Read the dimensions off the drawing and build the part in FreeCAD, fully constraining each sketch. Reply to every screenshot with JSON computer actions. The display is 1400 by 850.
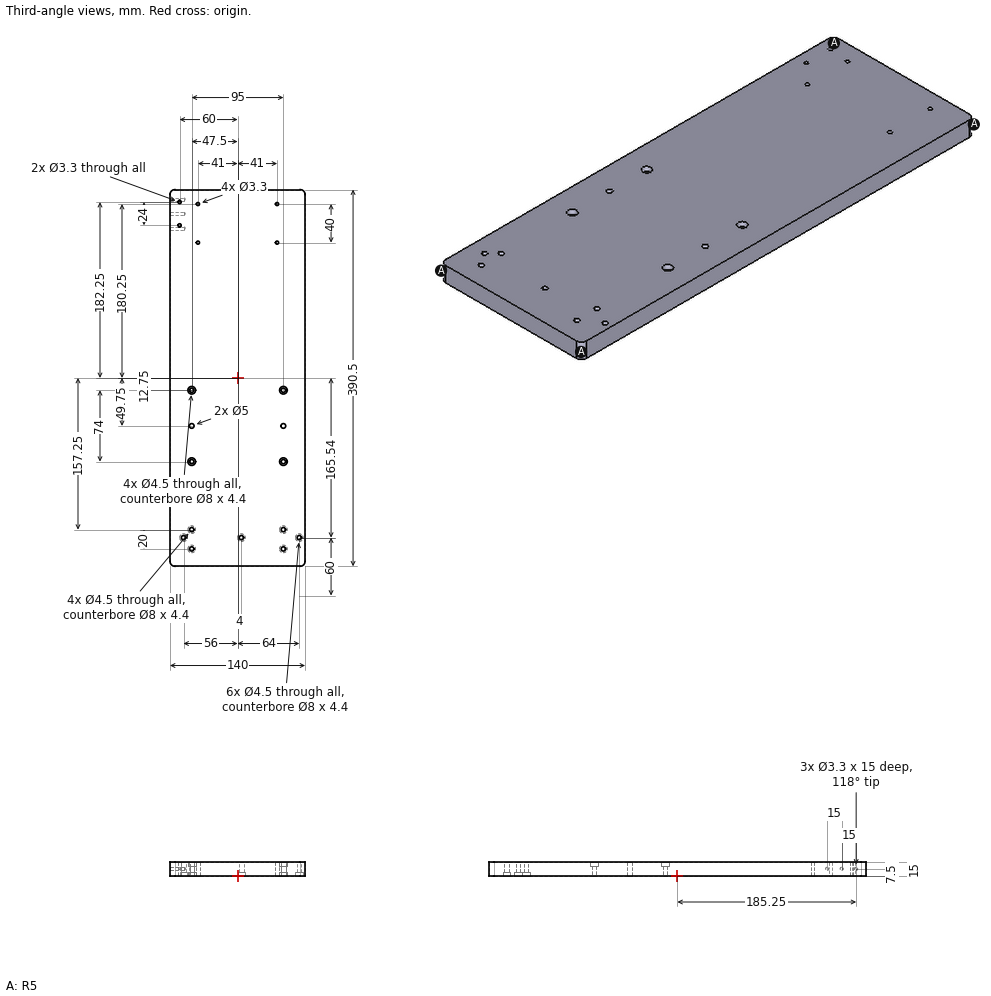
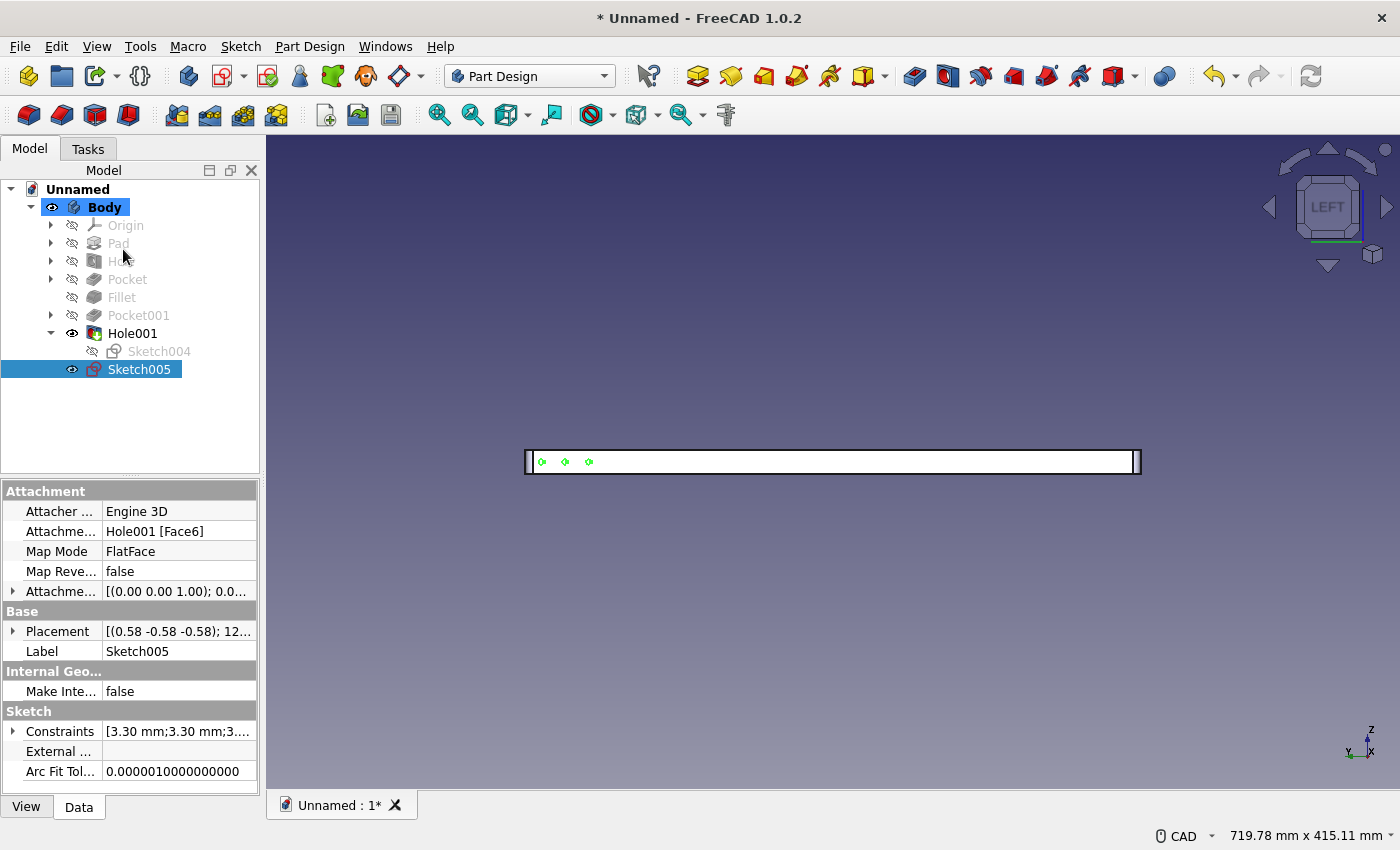
{"action": "left_click", "coordinate": [948, 76]}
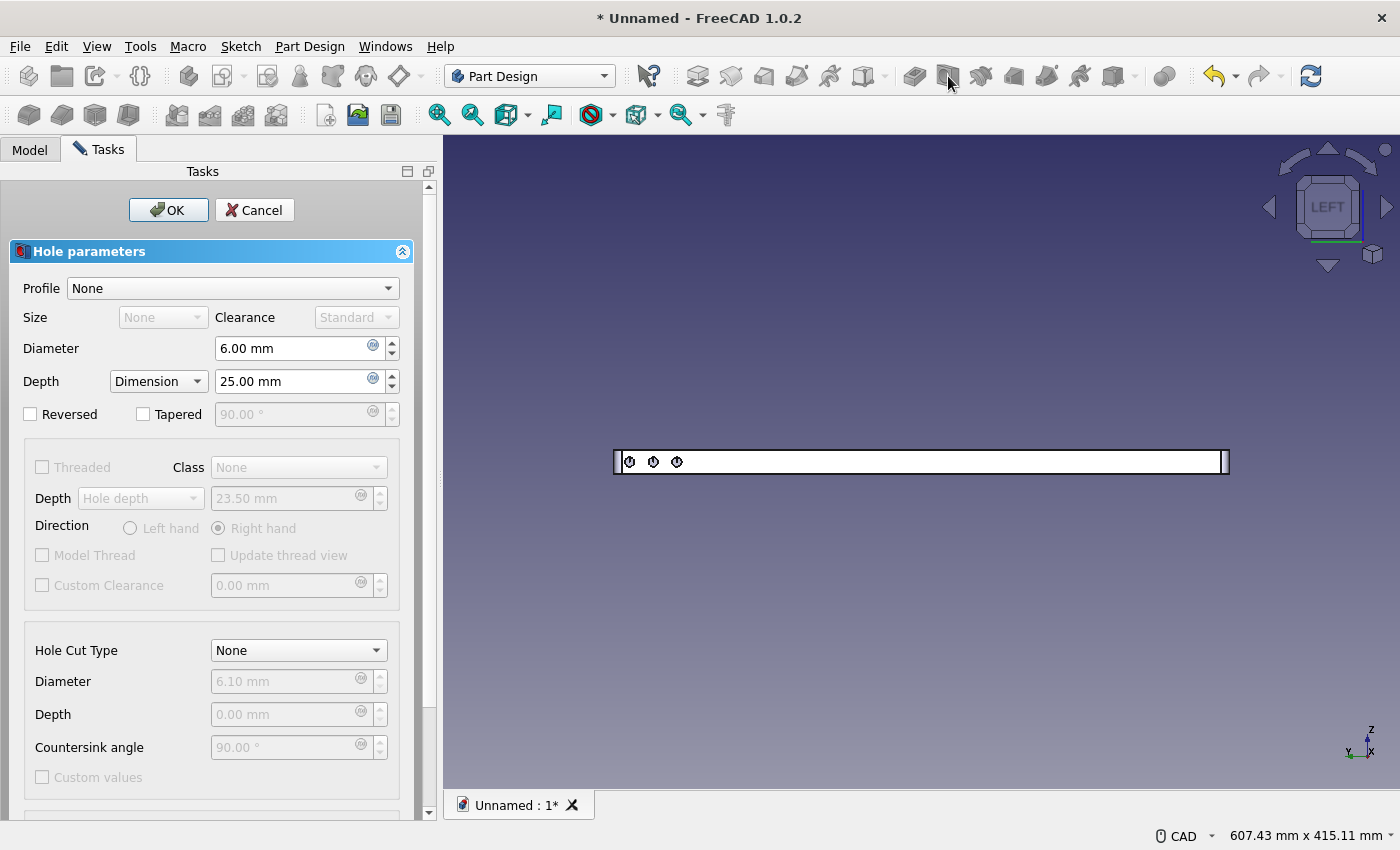
{"action": "triple_click", "coordinate": [300, 348]}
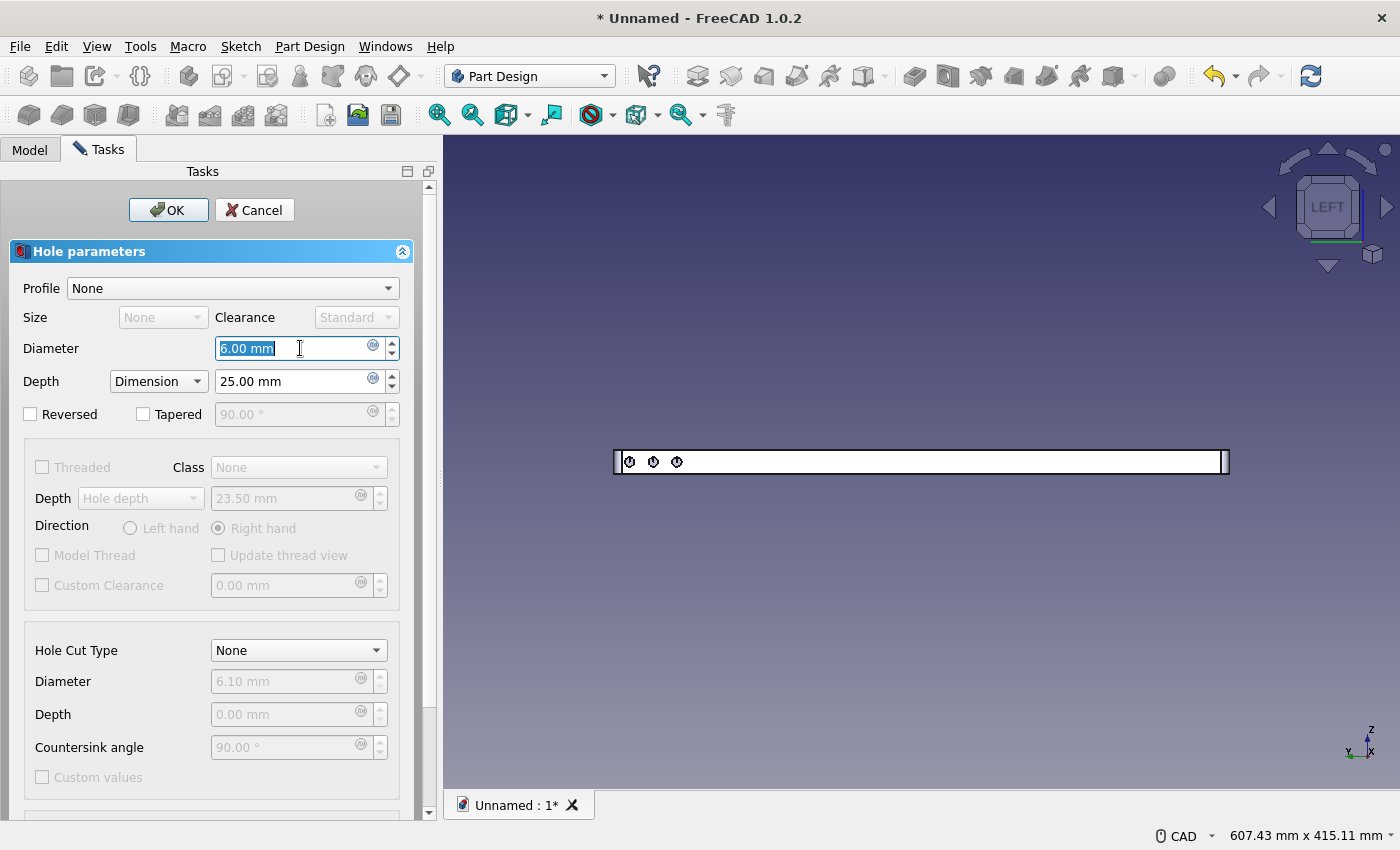
{"action": "type", "text": "3.3"}
{"action": "key", "text": "Tab"}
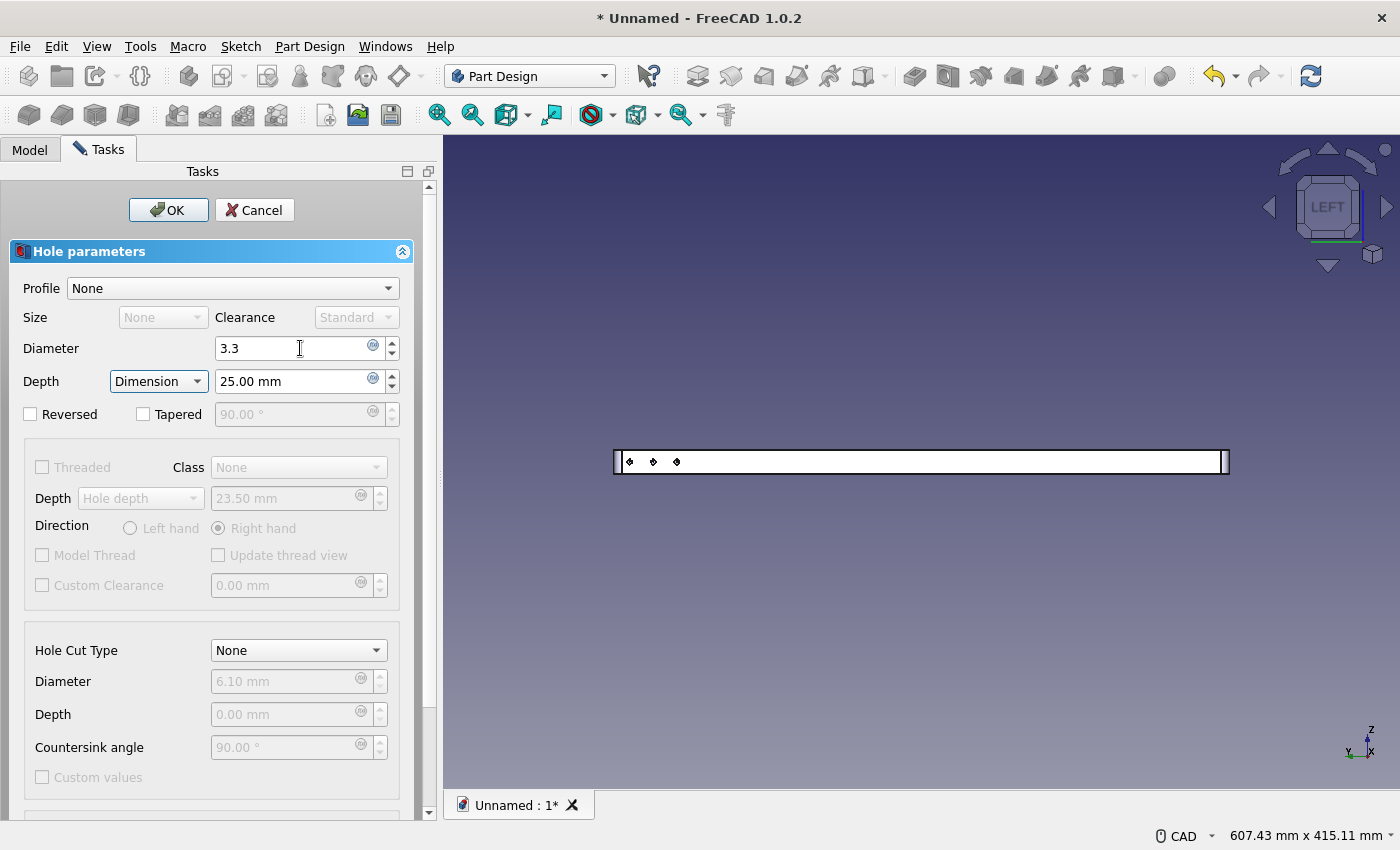
{"action": "triple_click", "coordinate": [300, 382]}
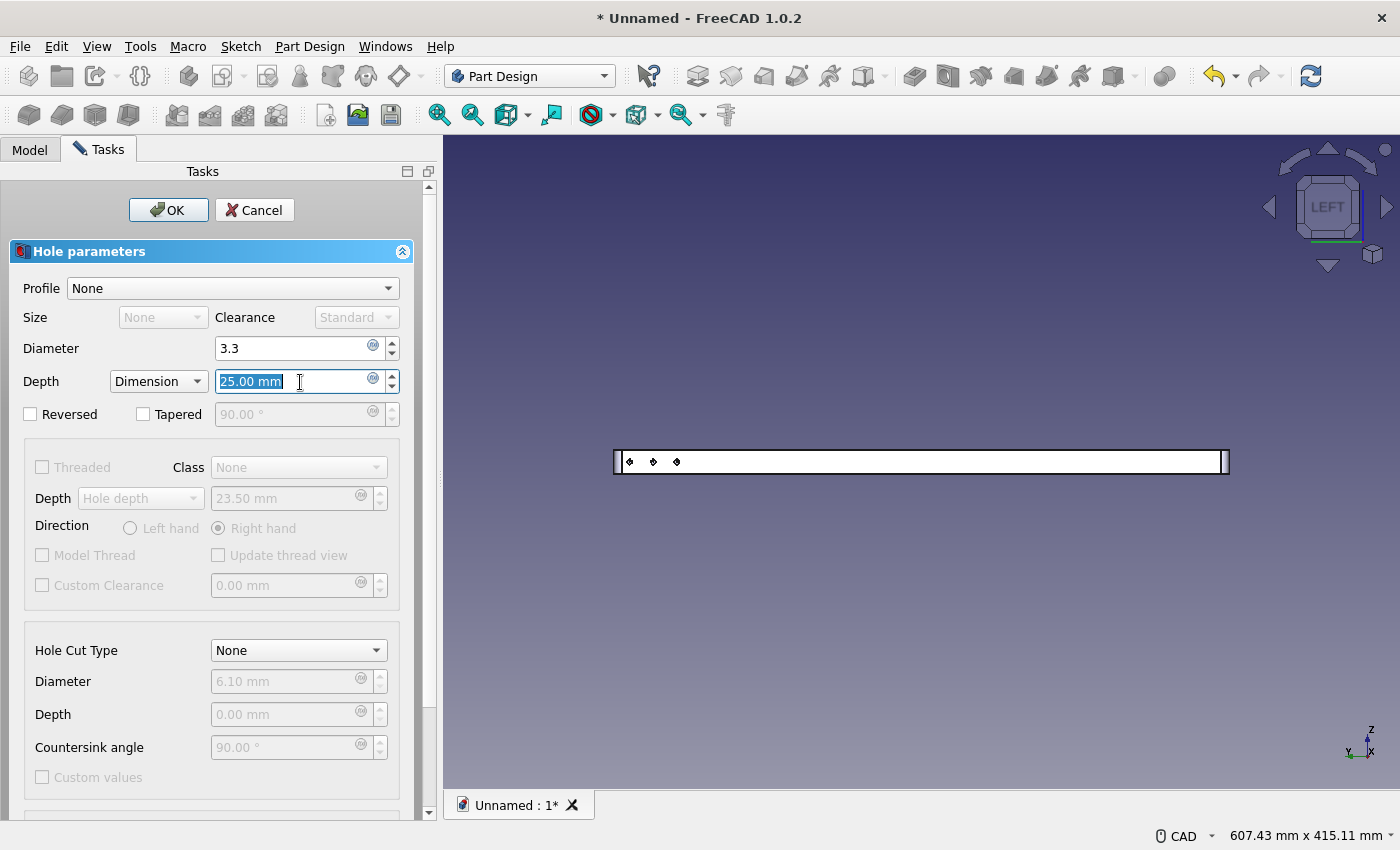
{"action": "type", "text": "15"}
{"action": "key", "text": "Tab"}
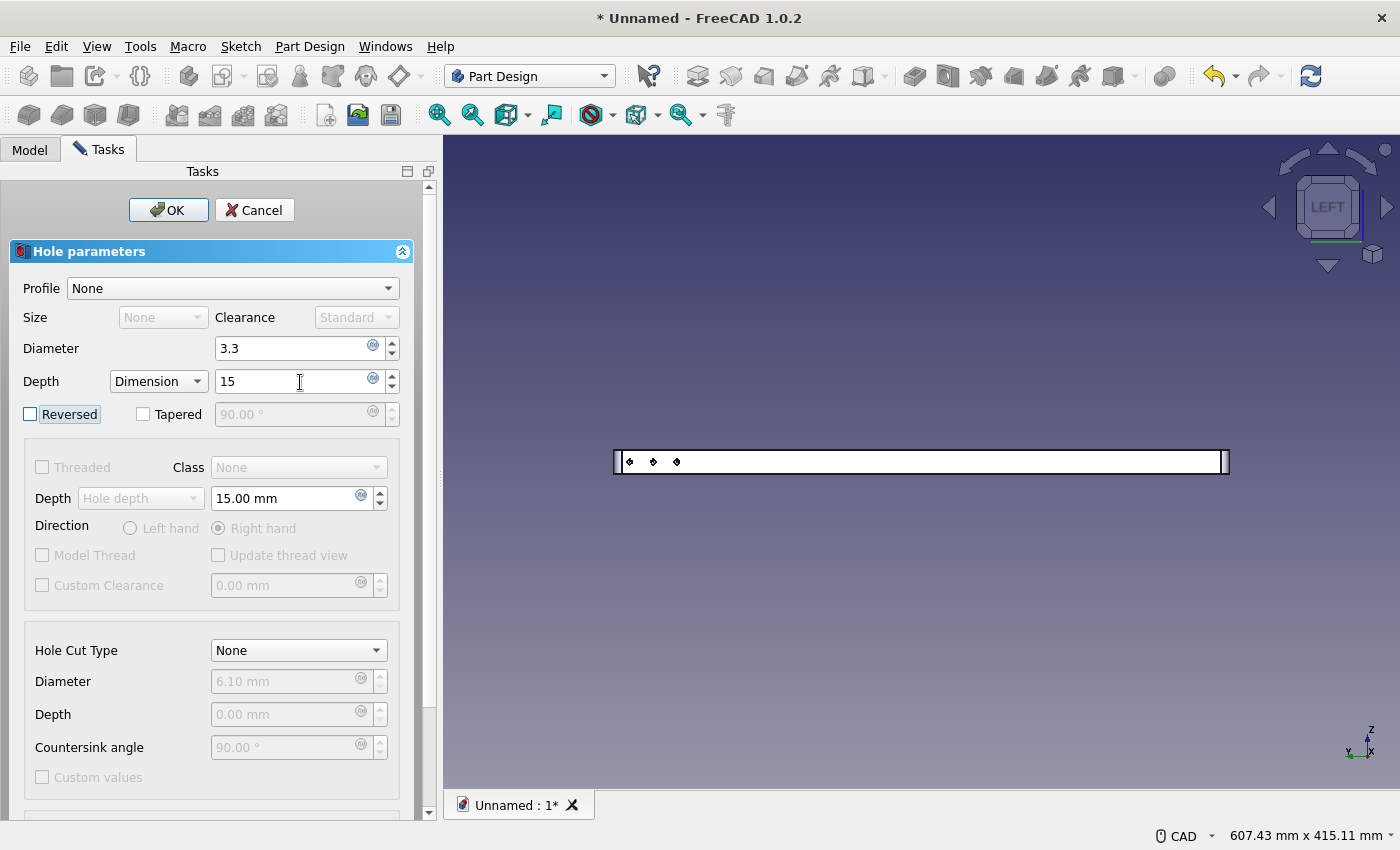
{"action": "left_click", "coordinate": [169, 210]}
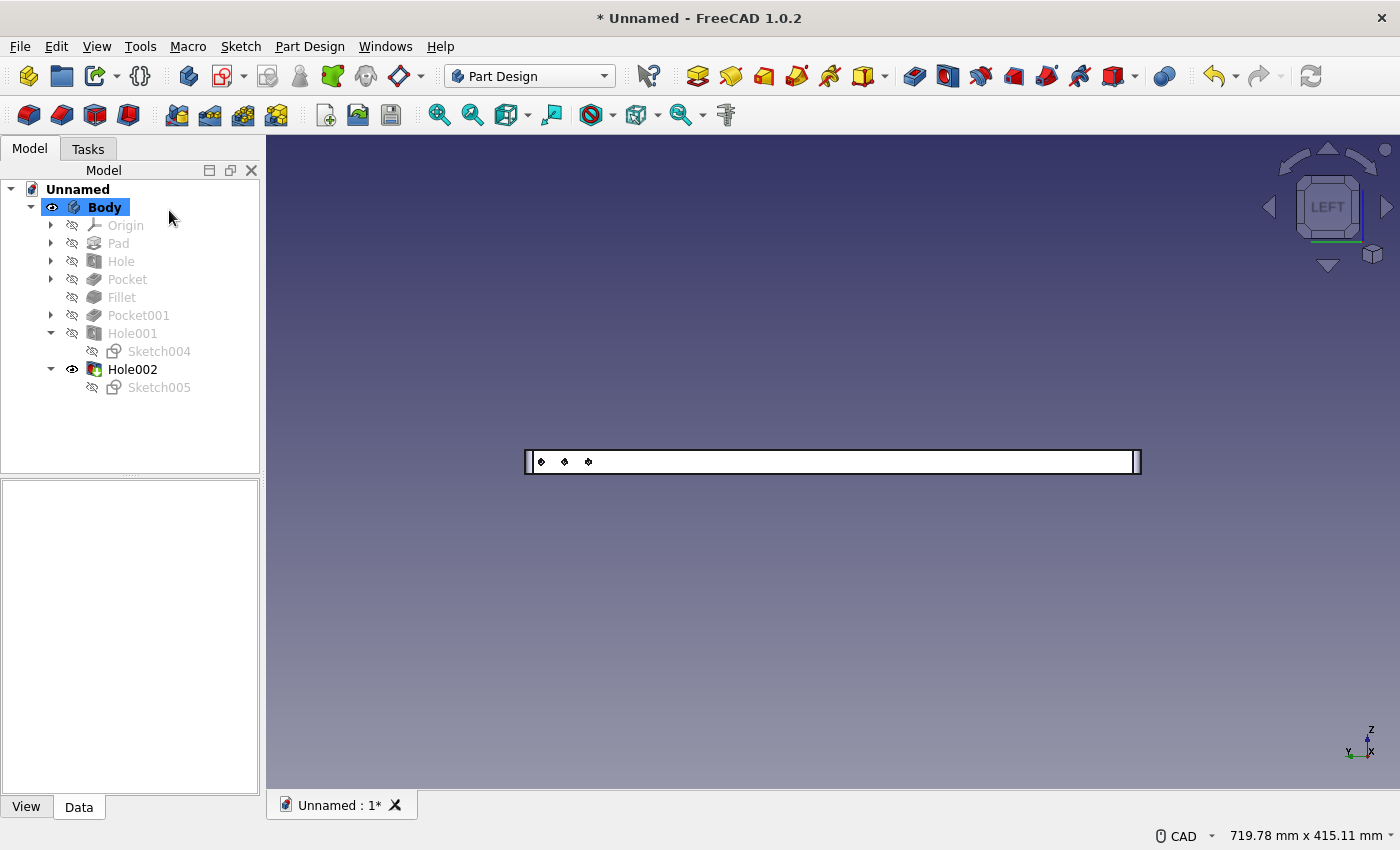
{"action": "key", "text": "0"}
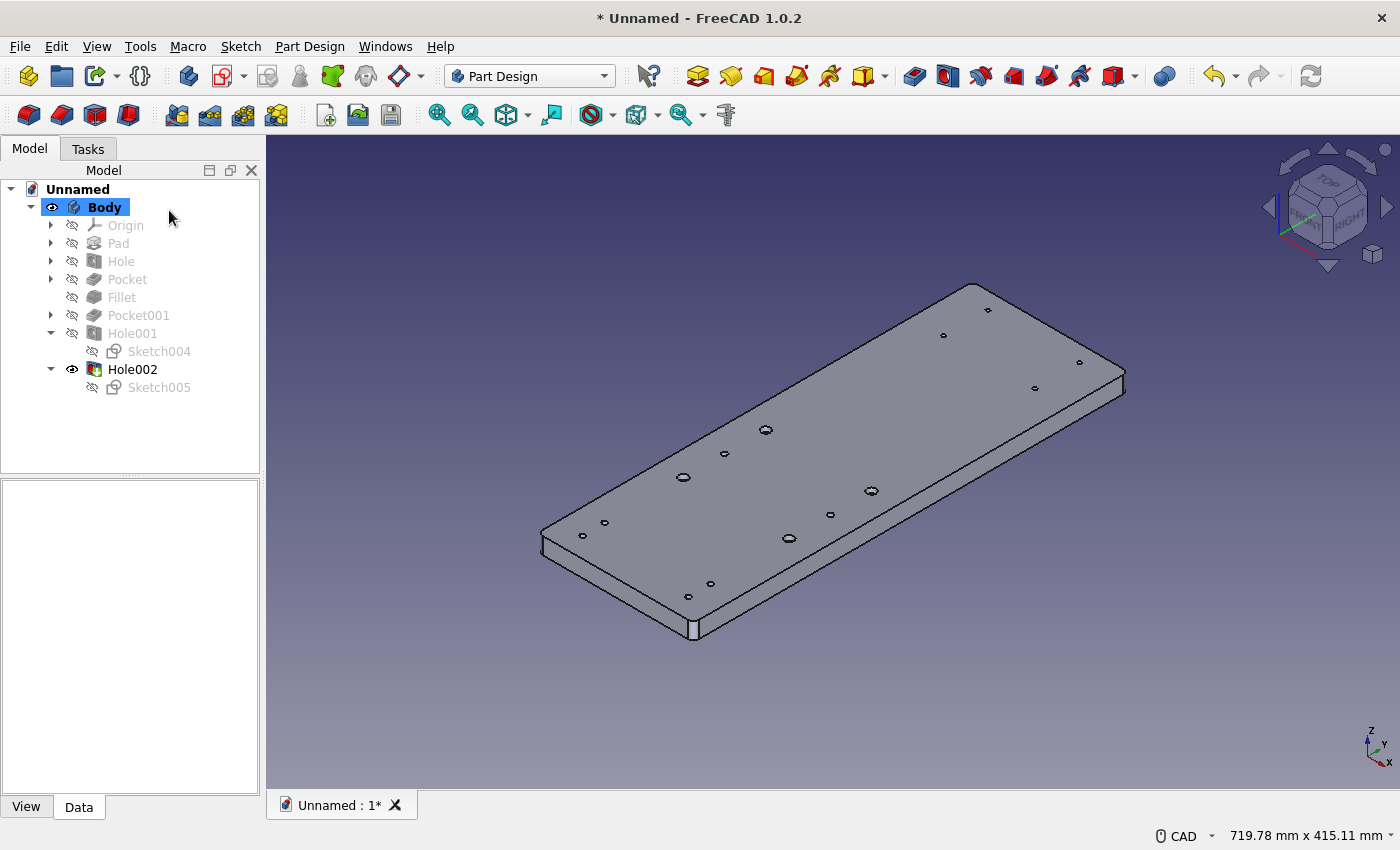
{"action": "left_click", "coordinate": [895, 415]}